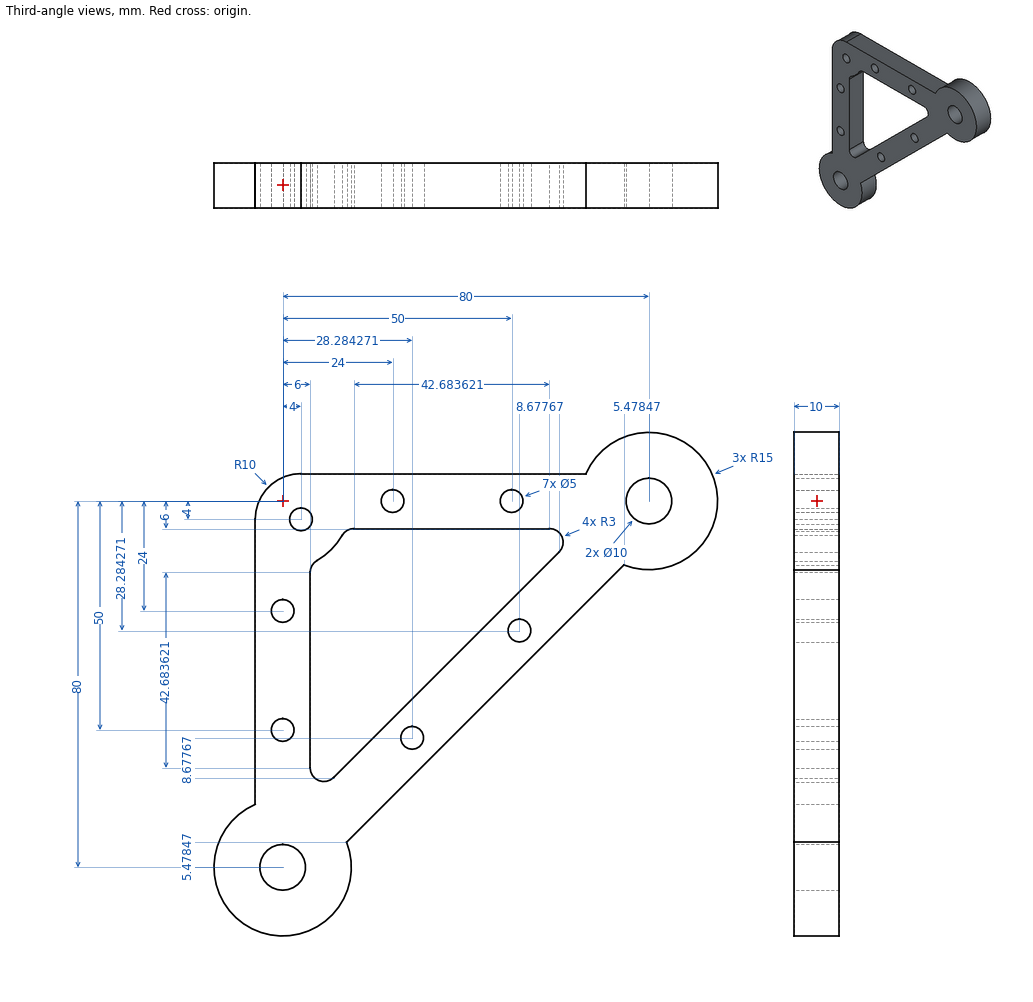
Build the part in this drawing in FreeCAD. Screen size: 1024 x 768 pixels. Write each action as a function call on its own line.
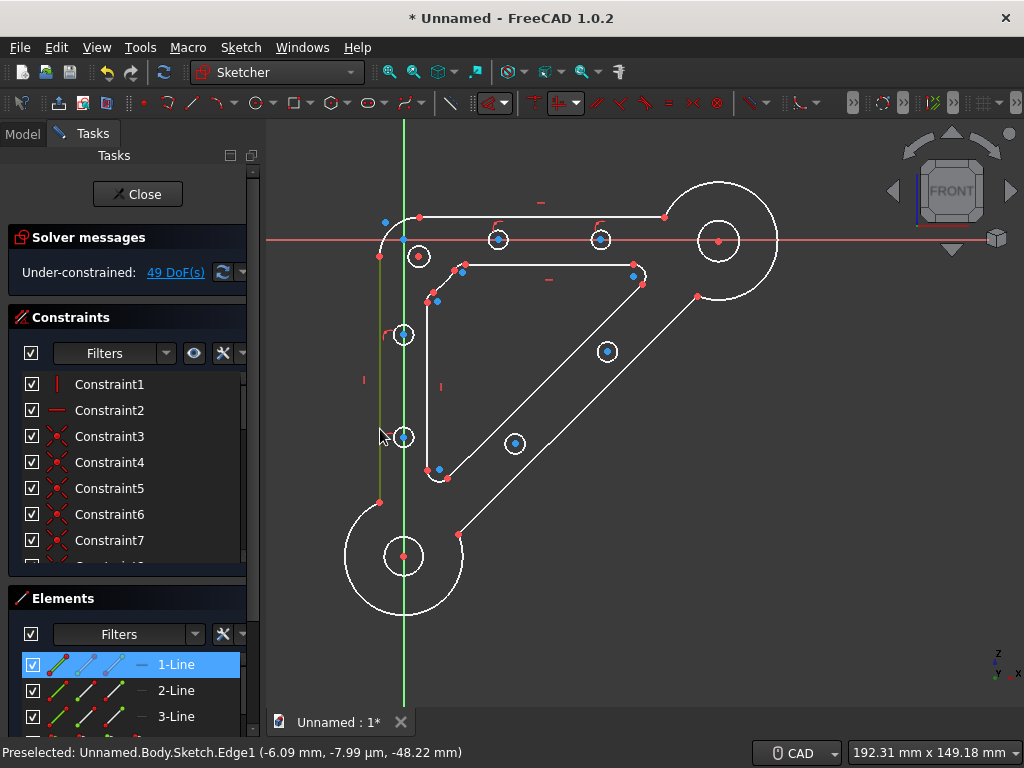
click(401, 222)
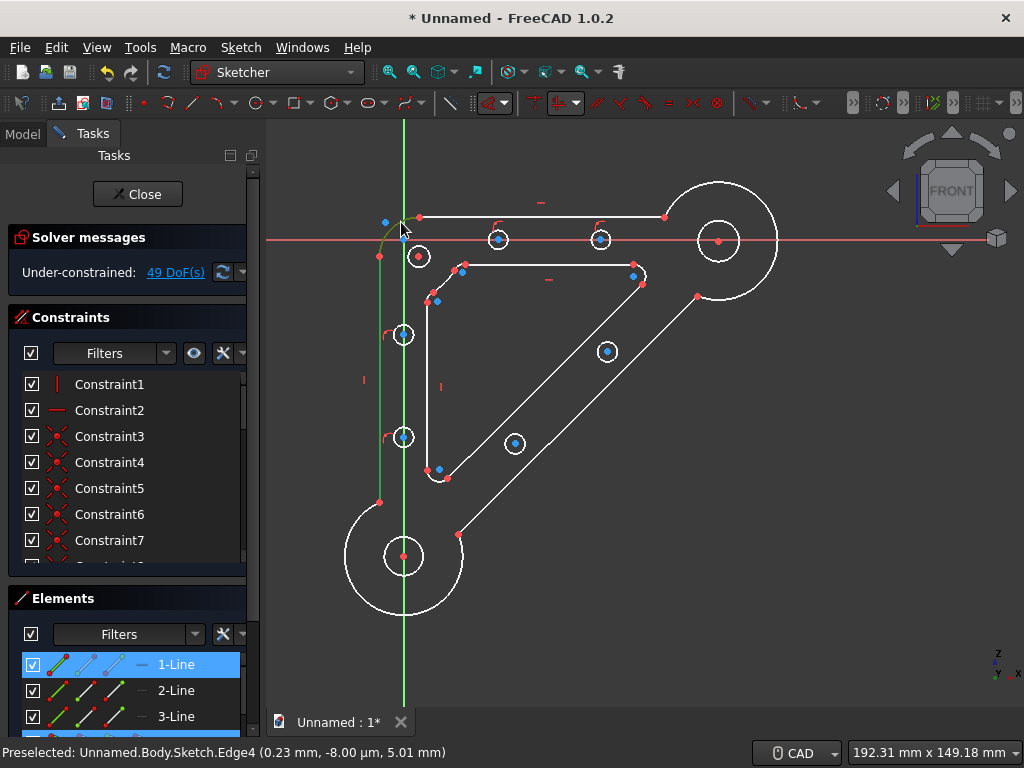
click(646, 104)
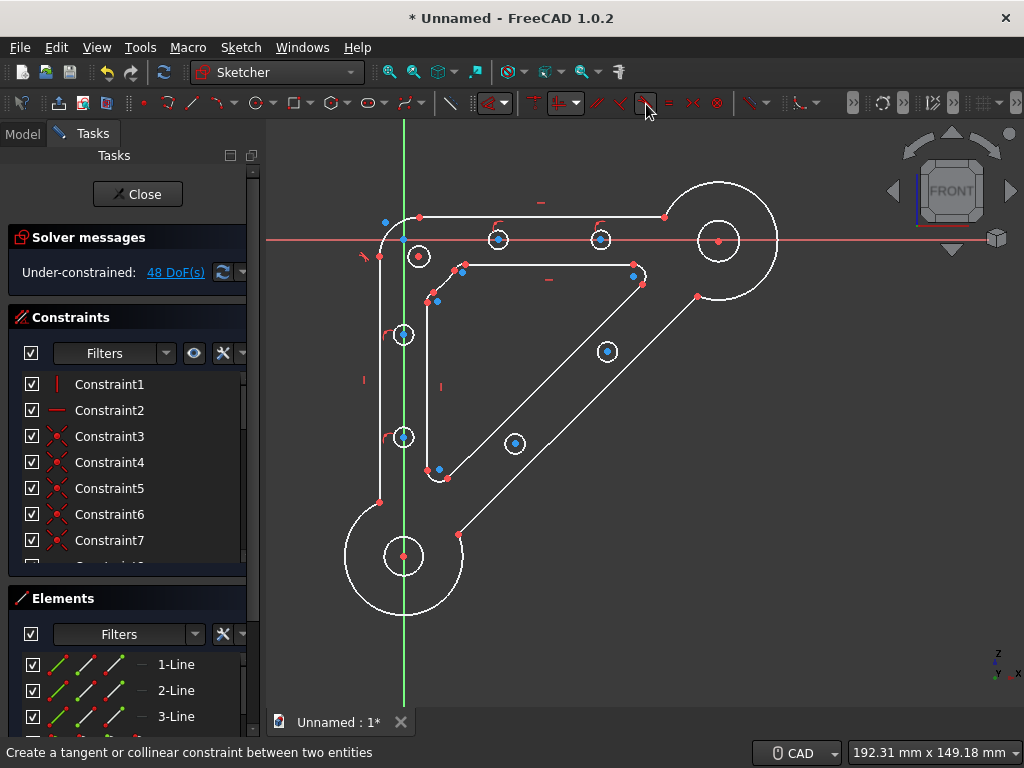
click(493, 217)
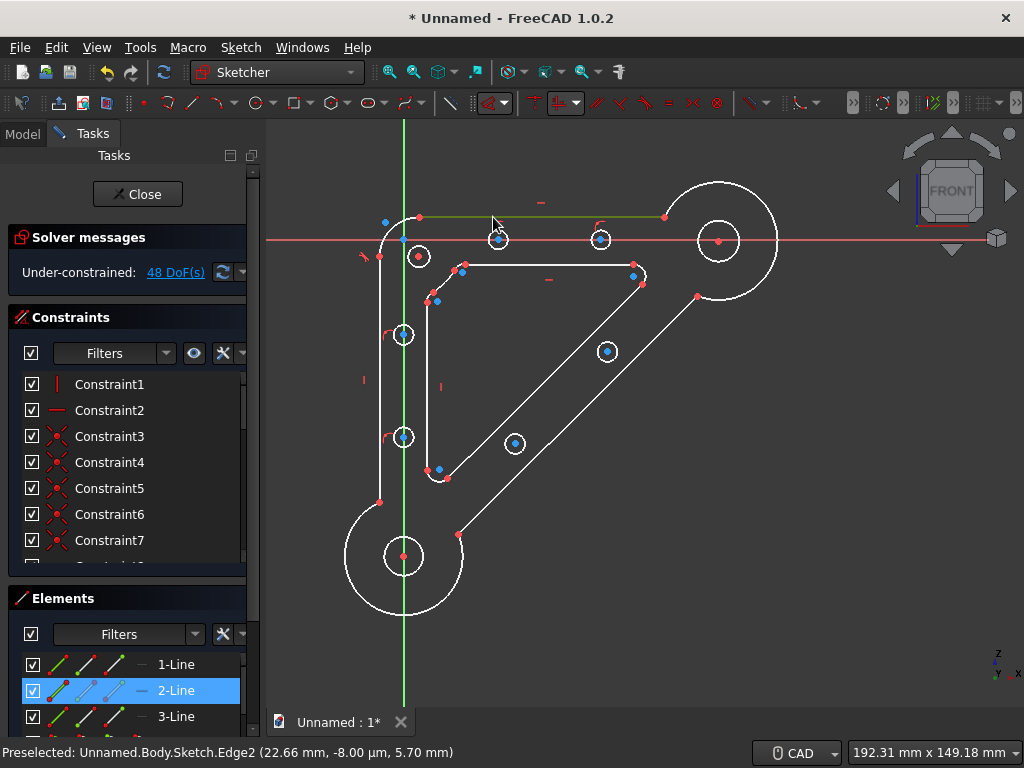
click(401, 222)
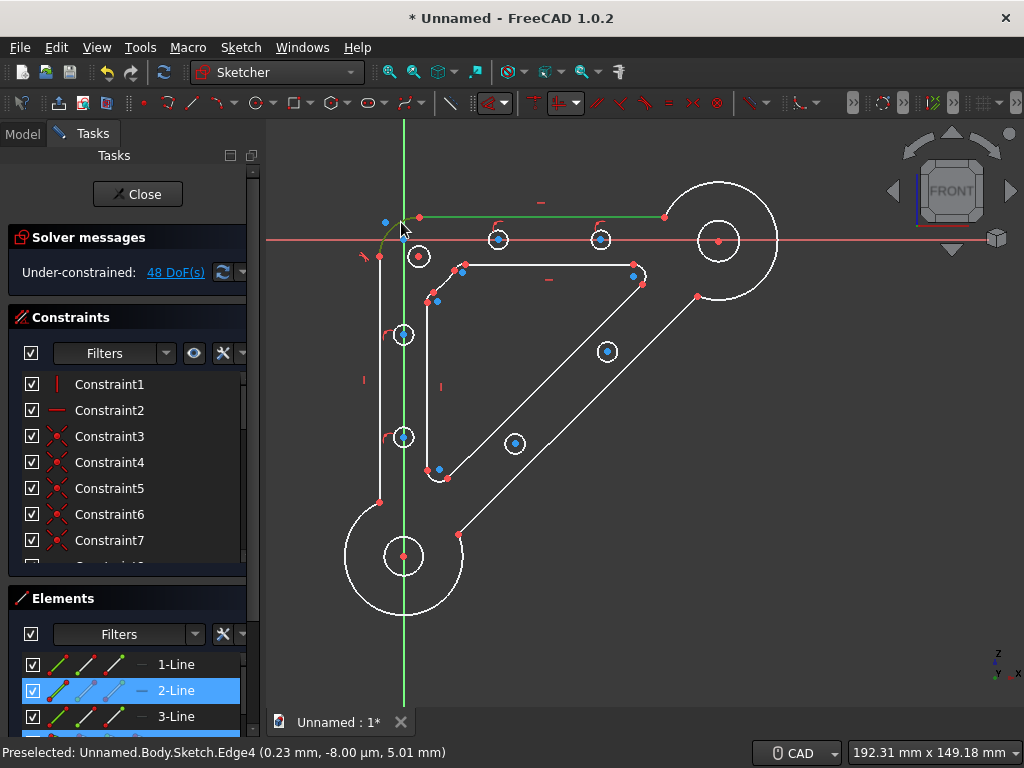
click(646, 104)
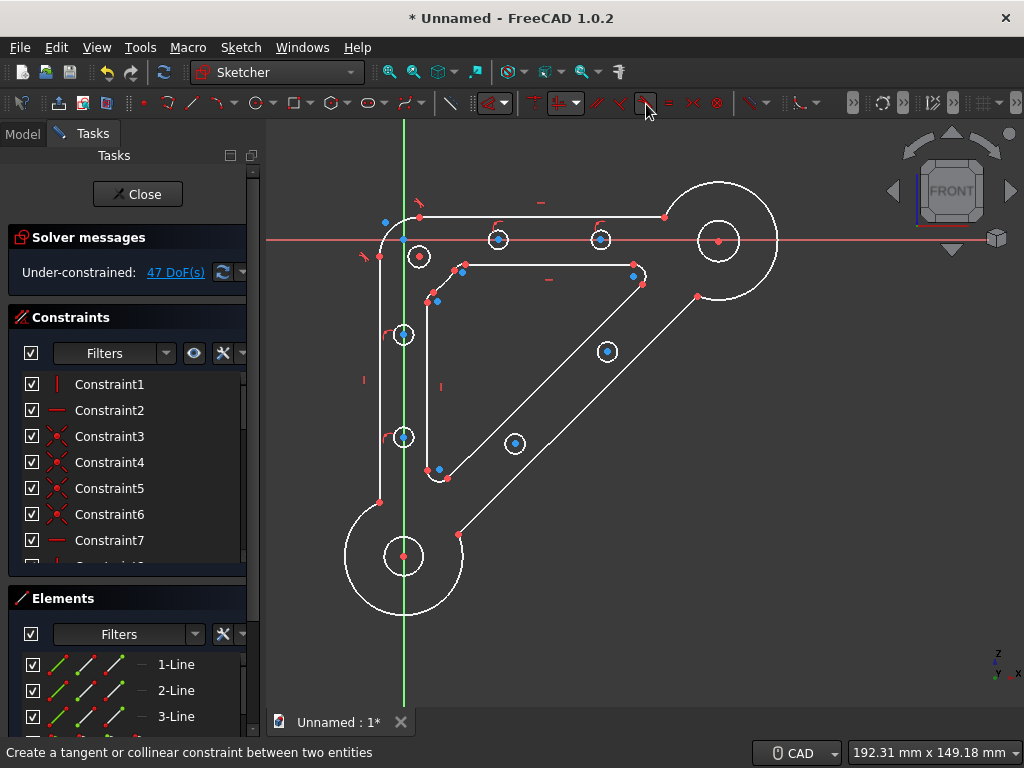
click(506, 421)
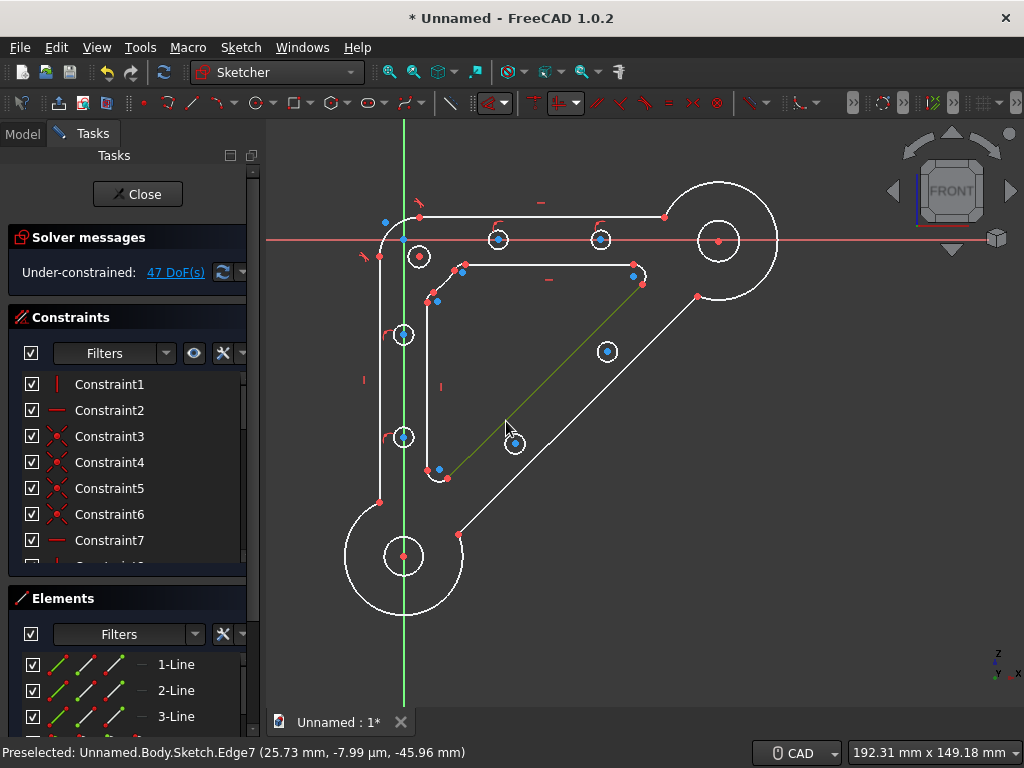
click(645, 272)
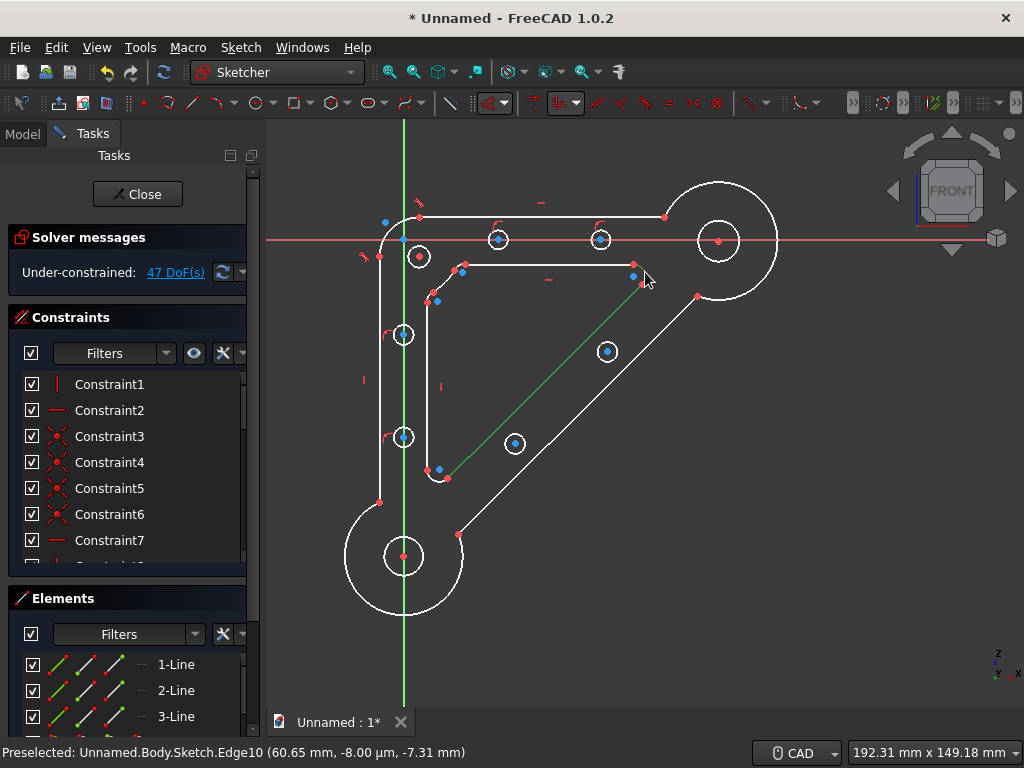
click(646, 104)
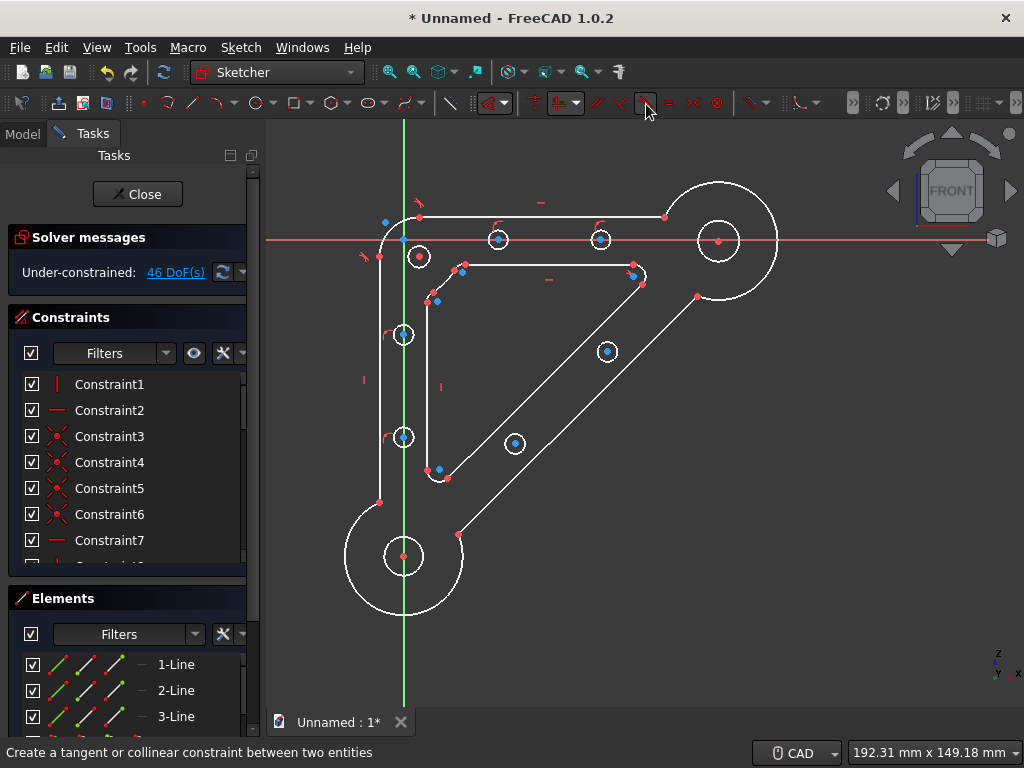
click(506, 421)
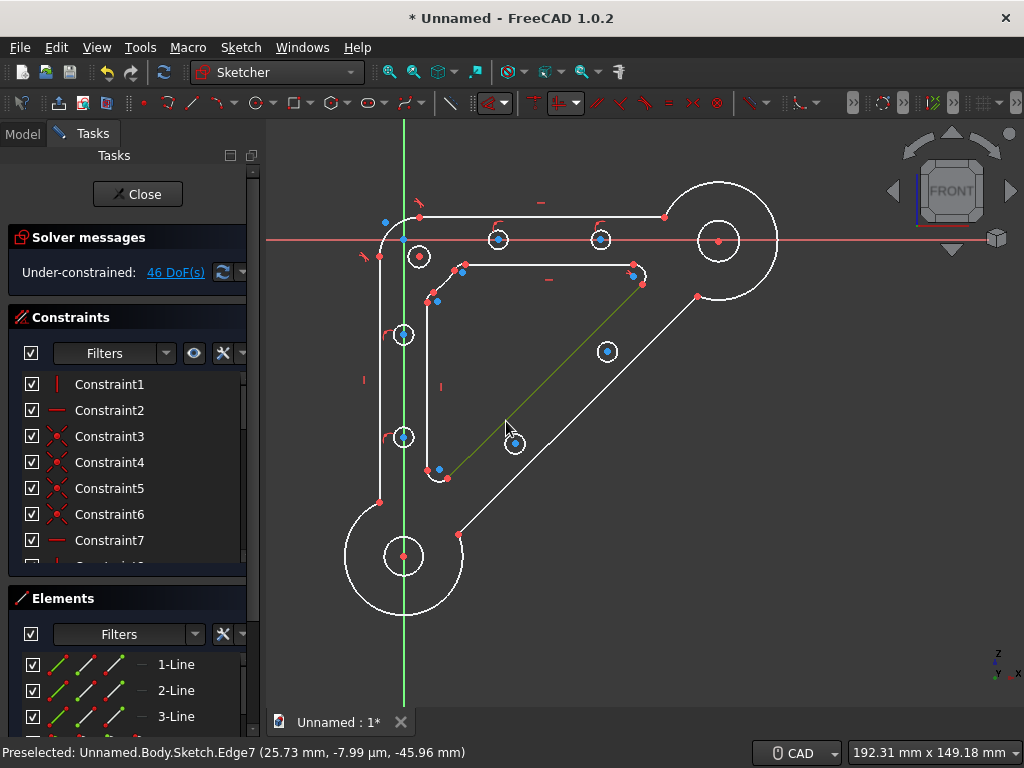
click(435, 481)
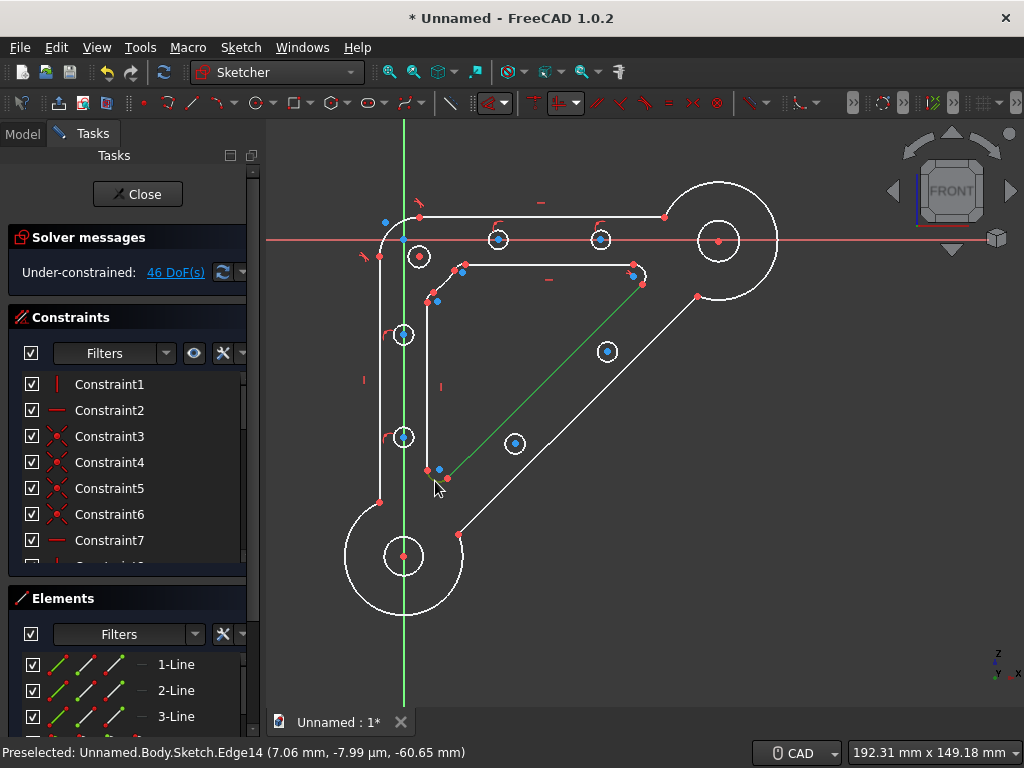
click(646, 104)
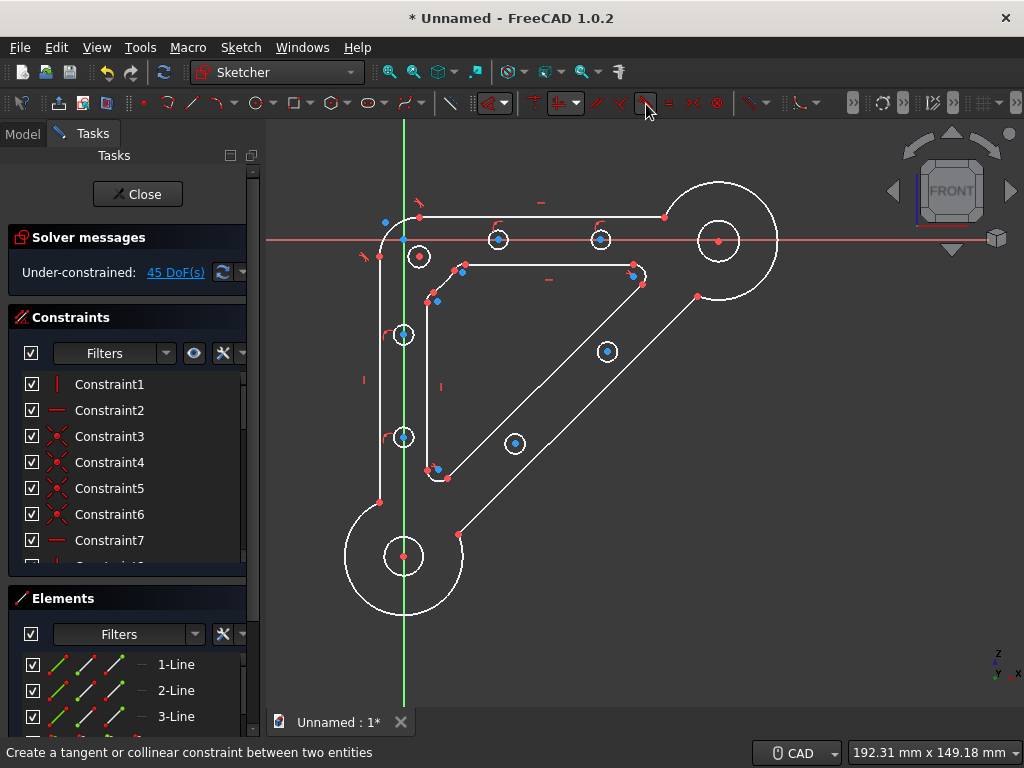
click(583, 265)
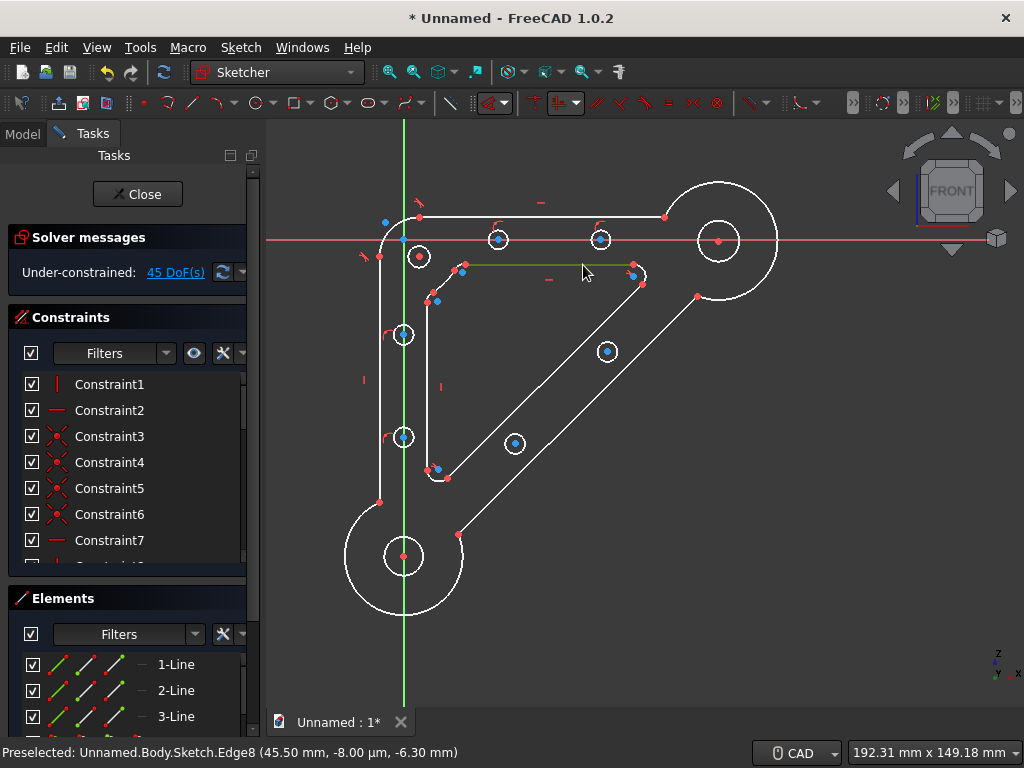
click(645, 272)